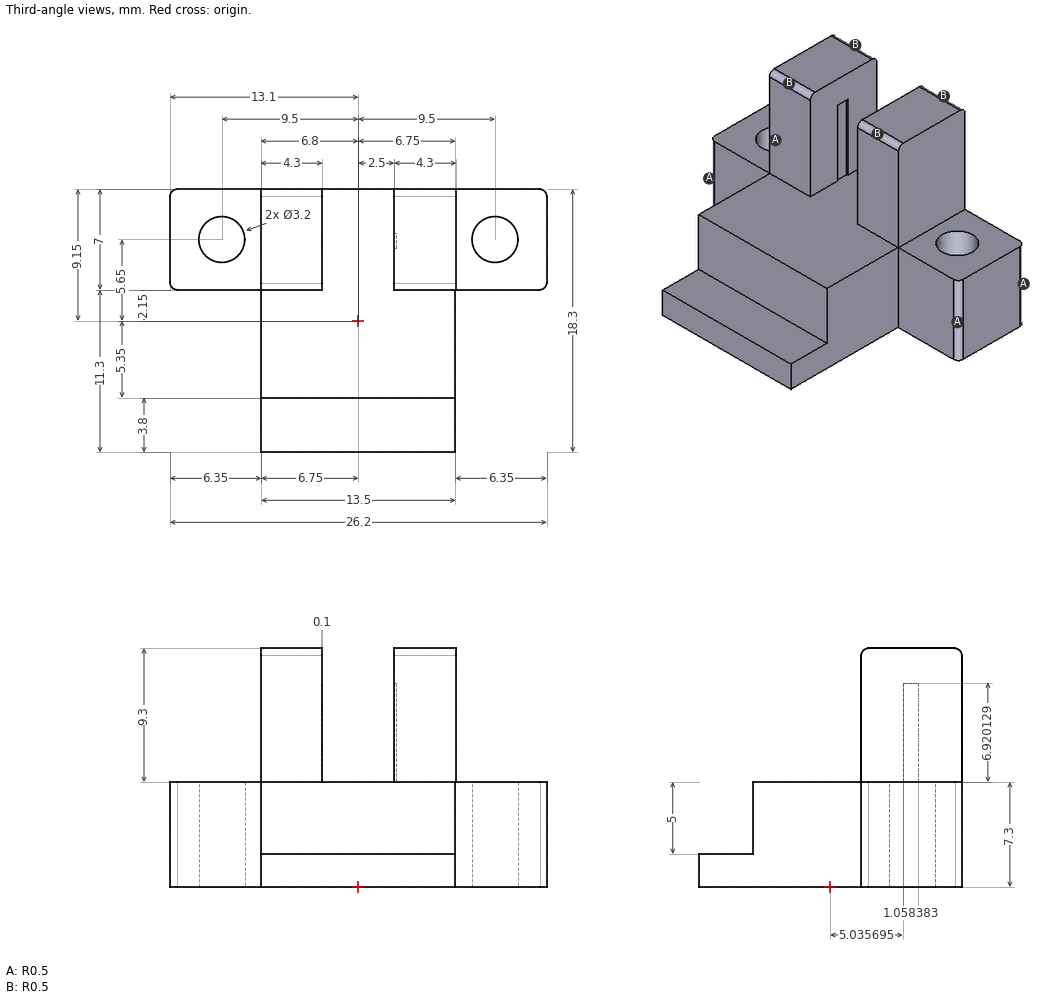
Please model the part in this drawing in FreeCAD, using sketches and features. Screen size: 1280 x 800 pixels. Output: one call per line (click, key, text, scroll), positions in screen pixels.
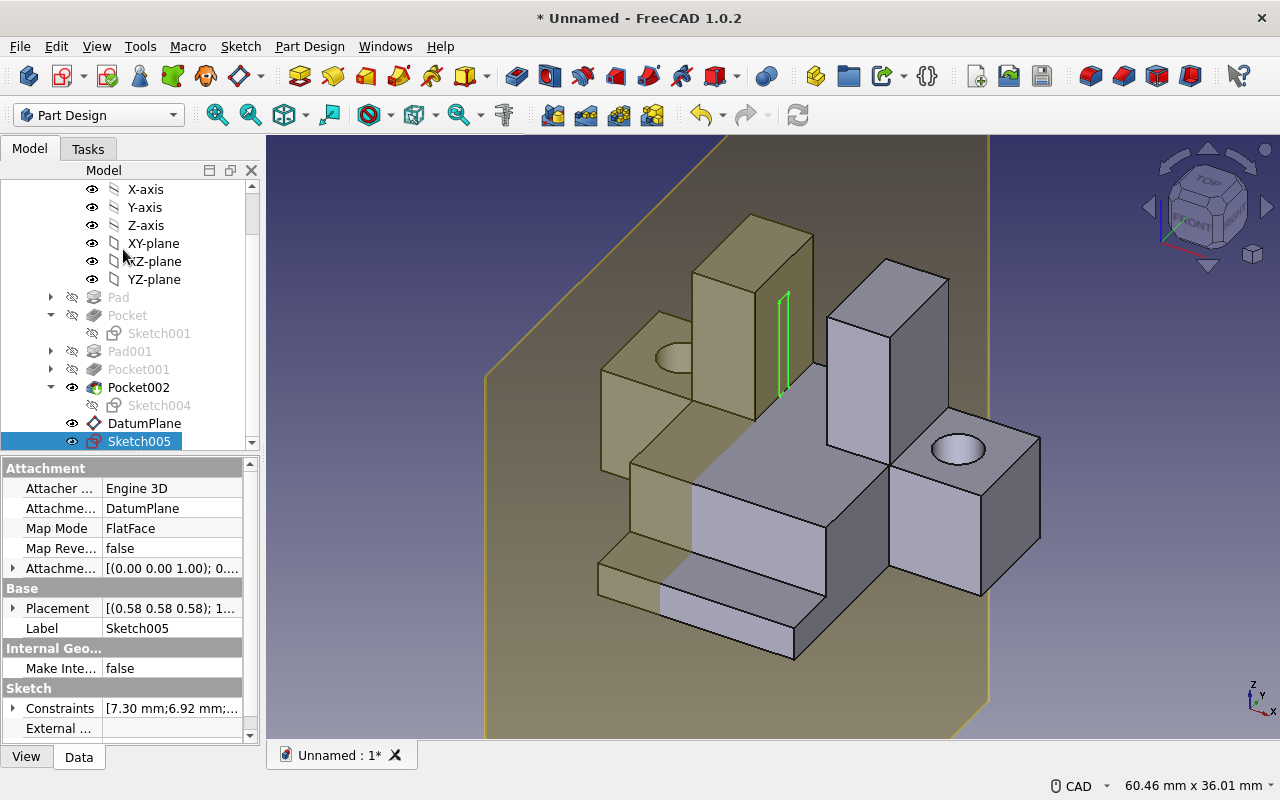
click(517, 76)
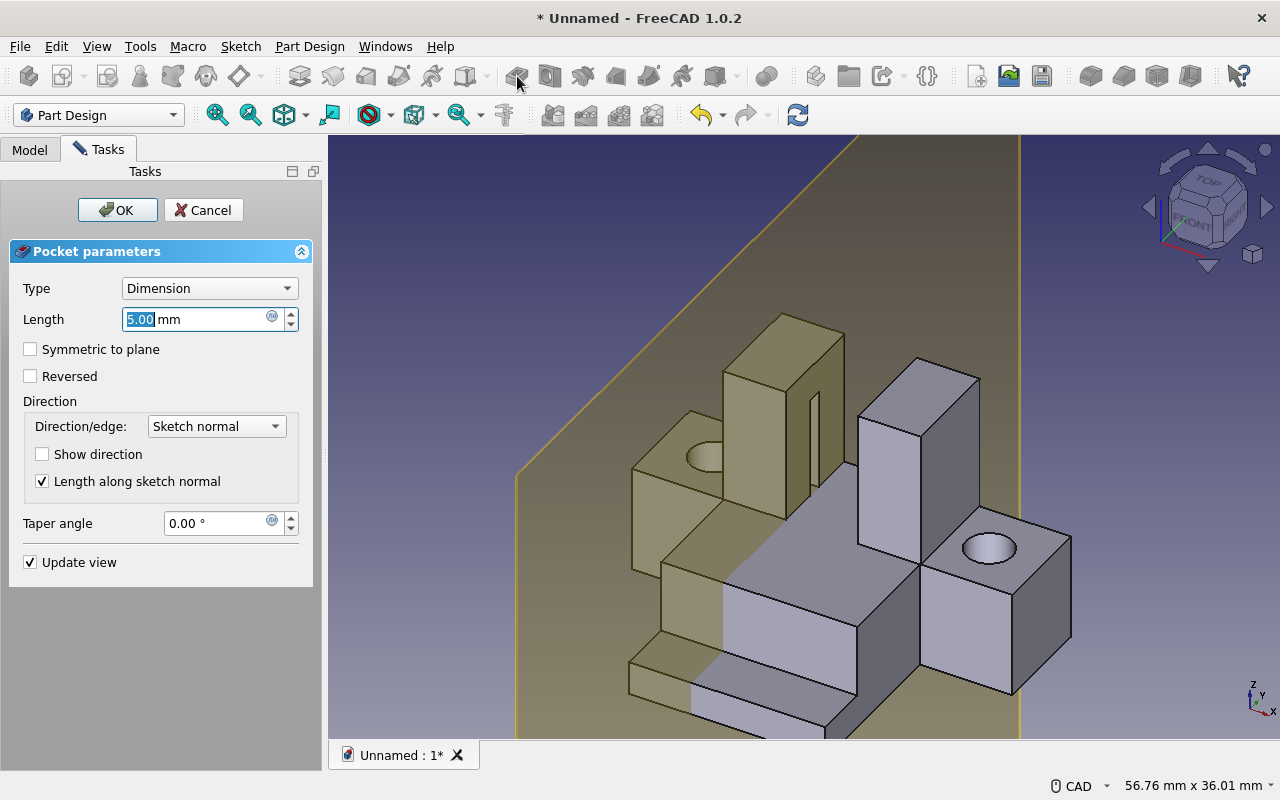
text(0.1)
key(Tab)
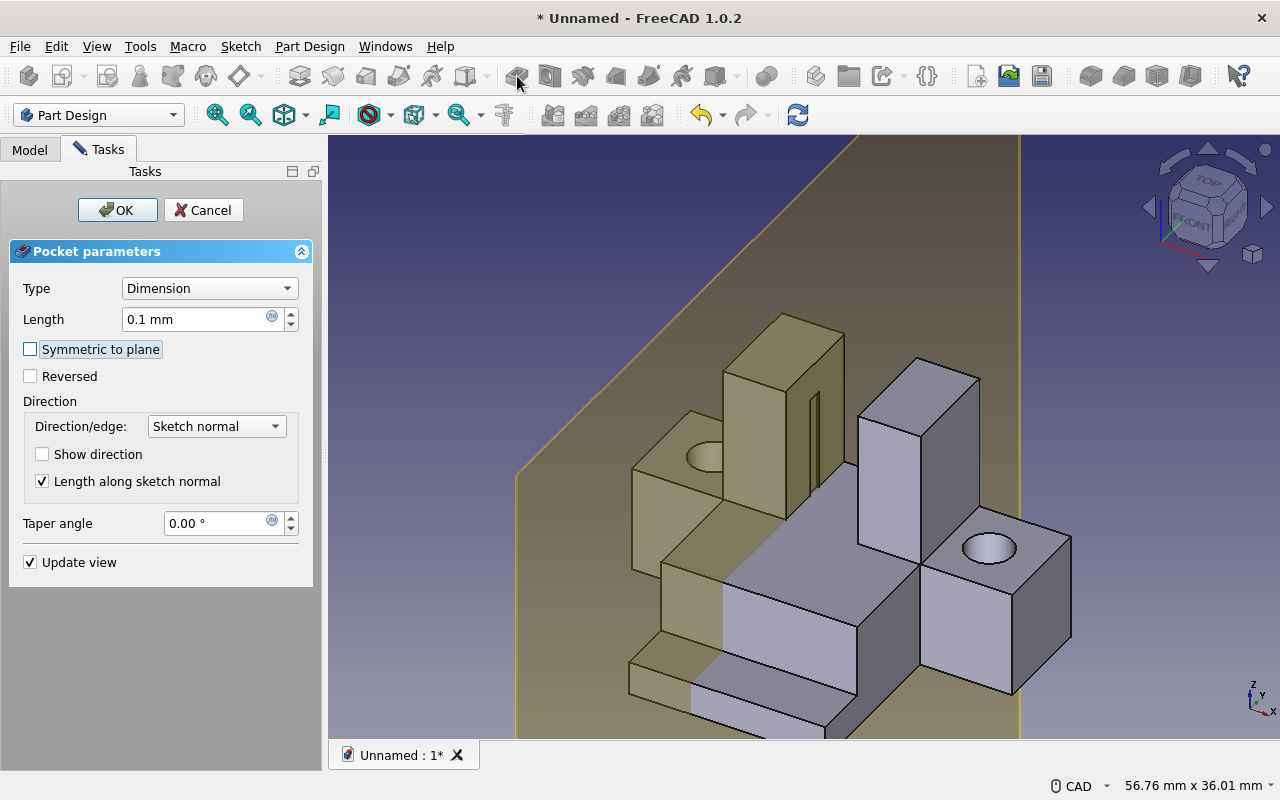
click(118, 210)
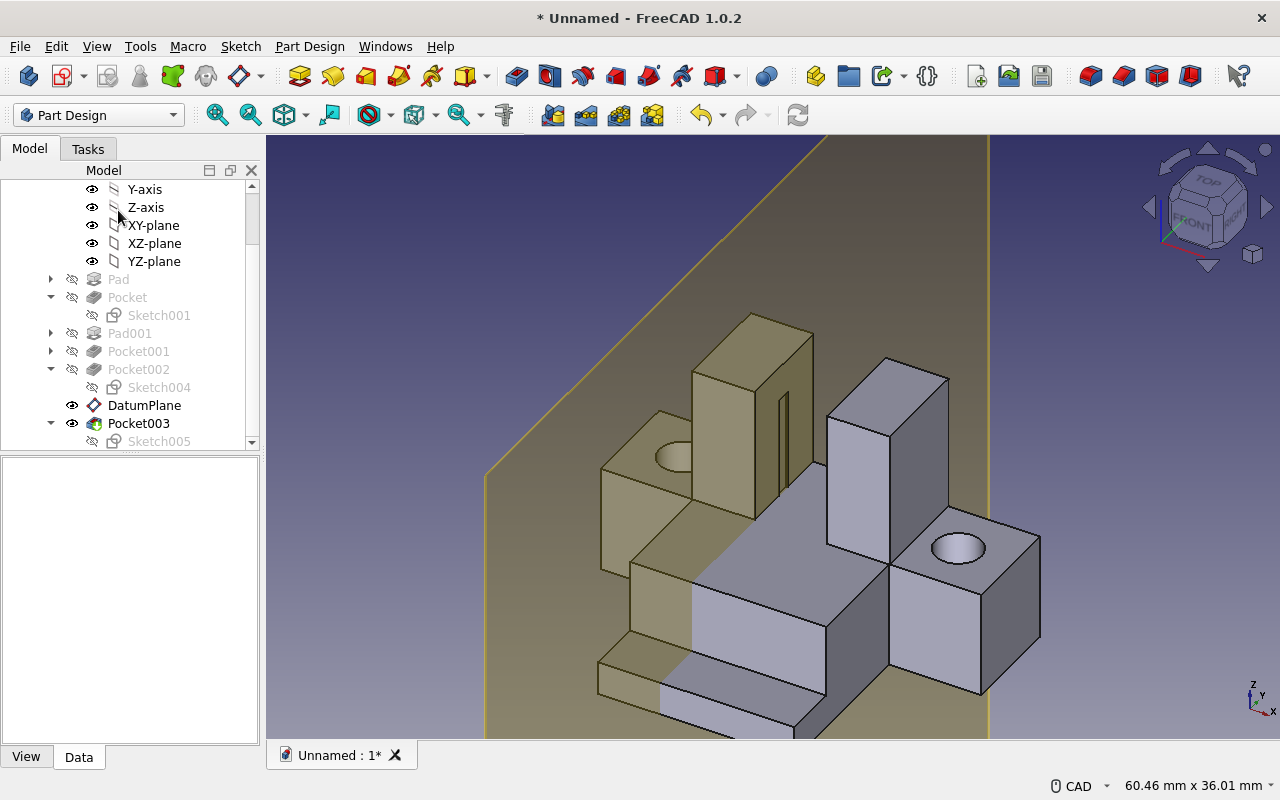
click(117, 405)
key(space)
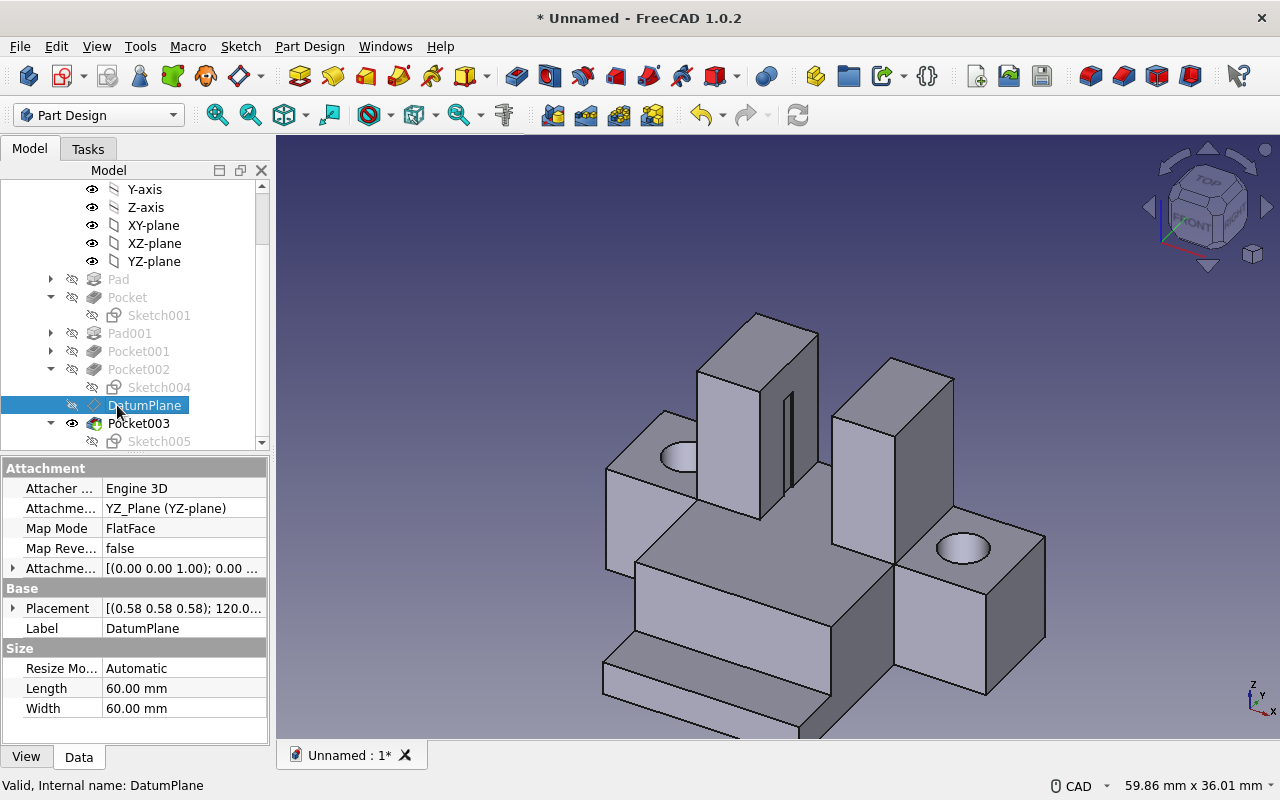
key(v)
key(f)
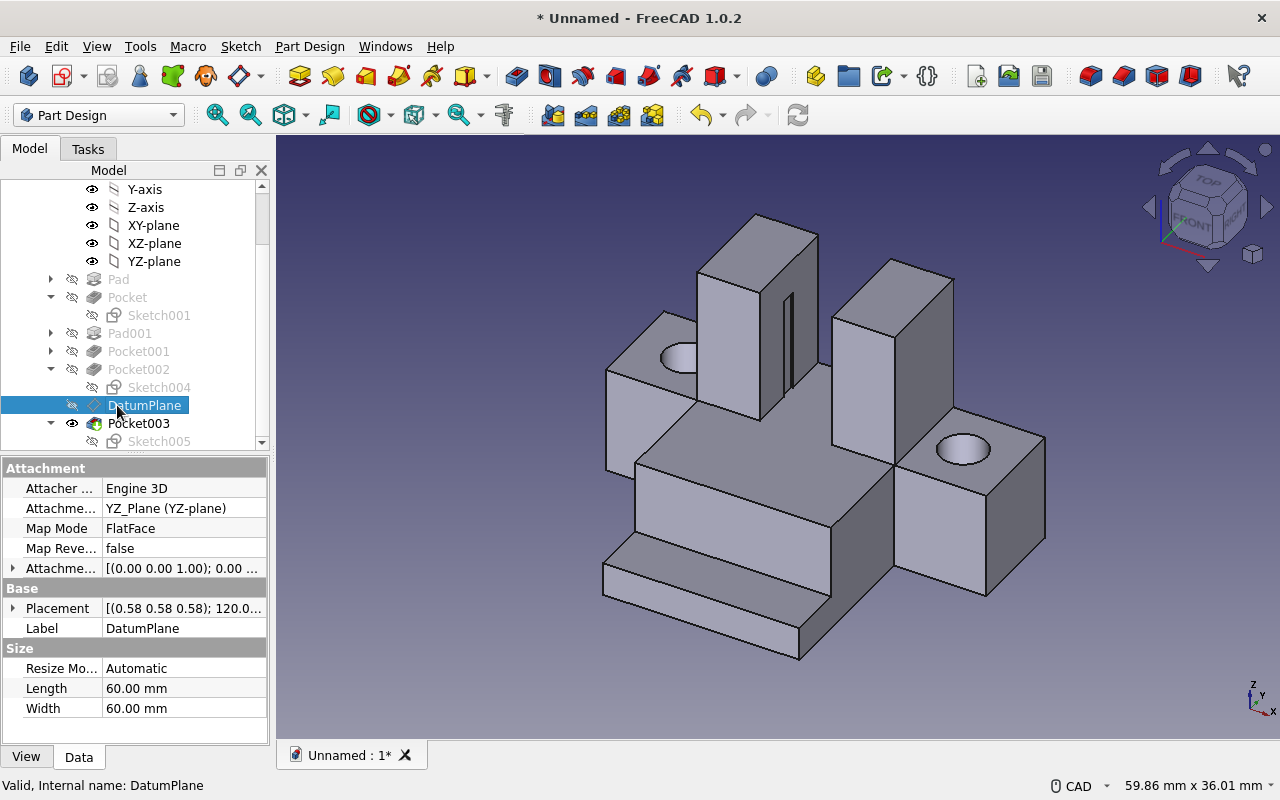
click(986, 545)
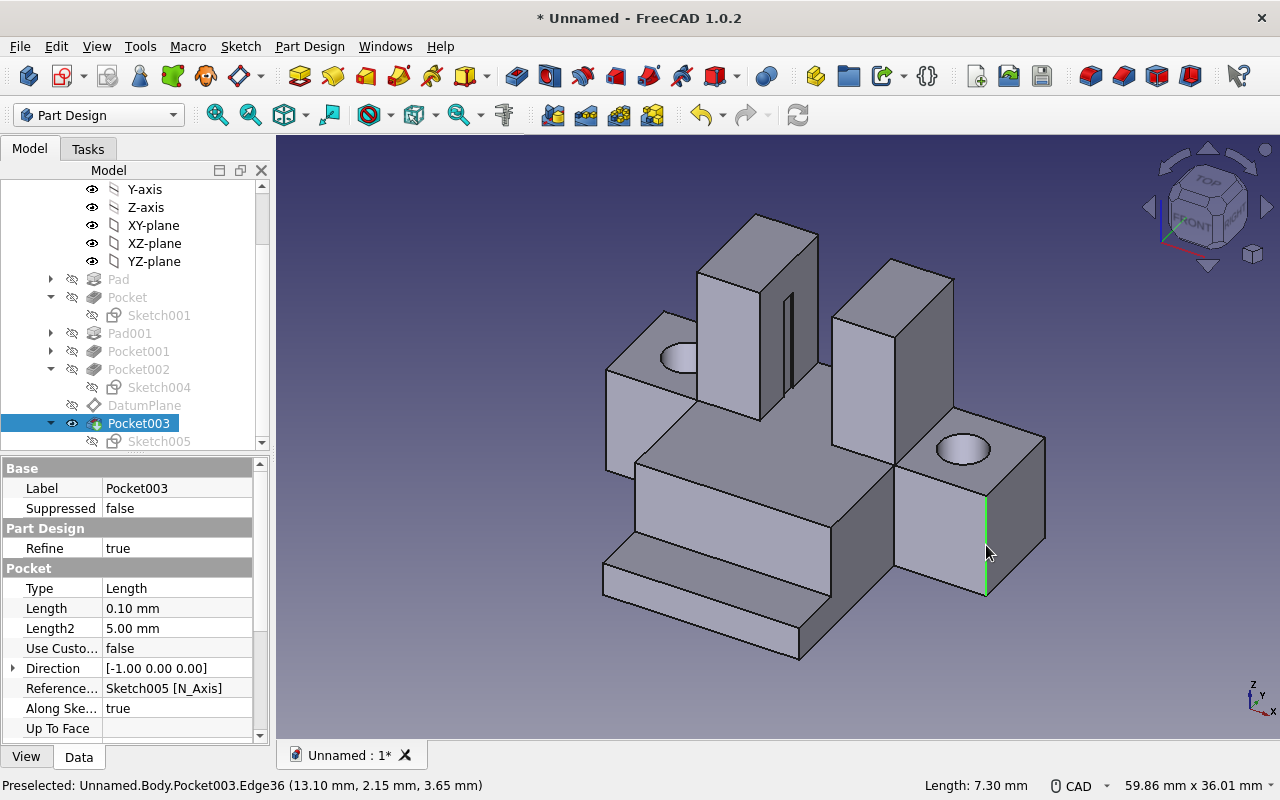
key(0)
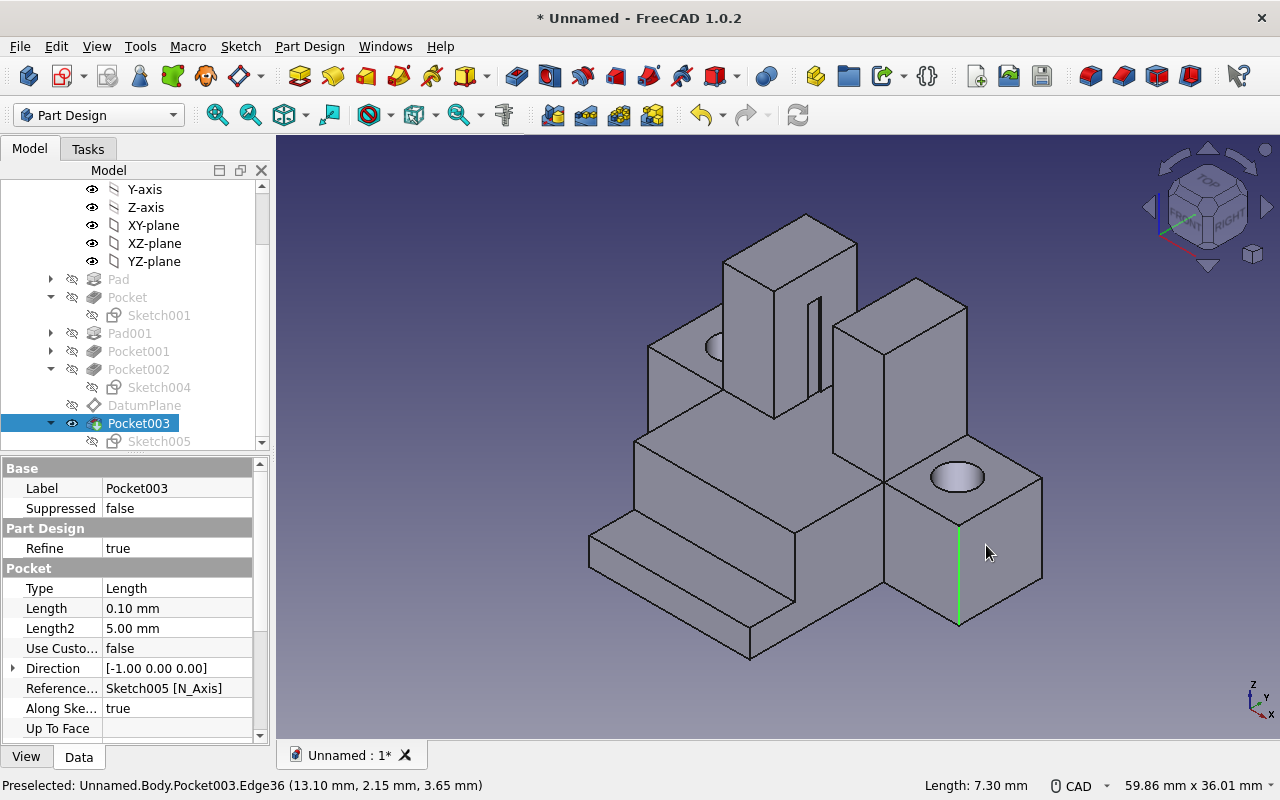
key(2)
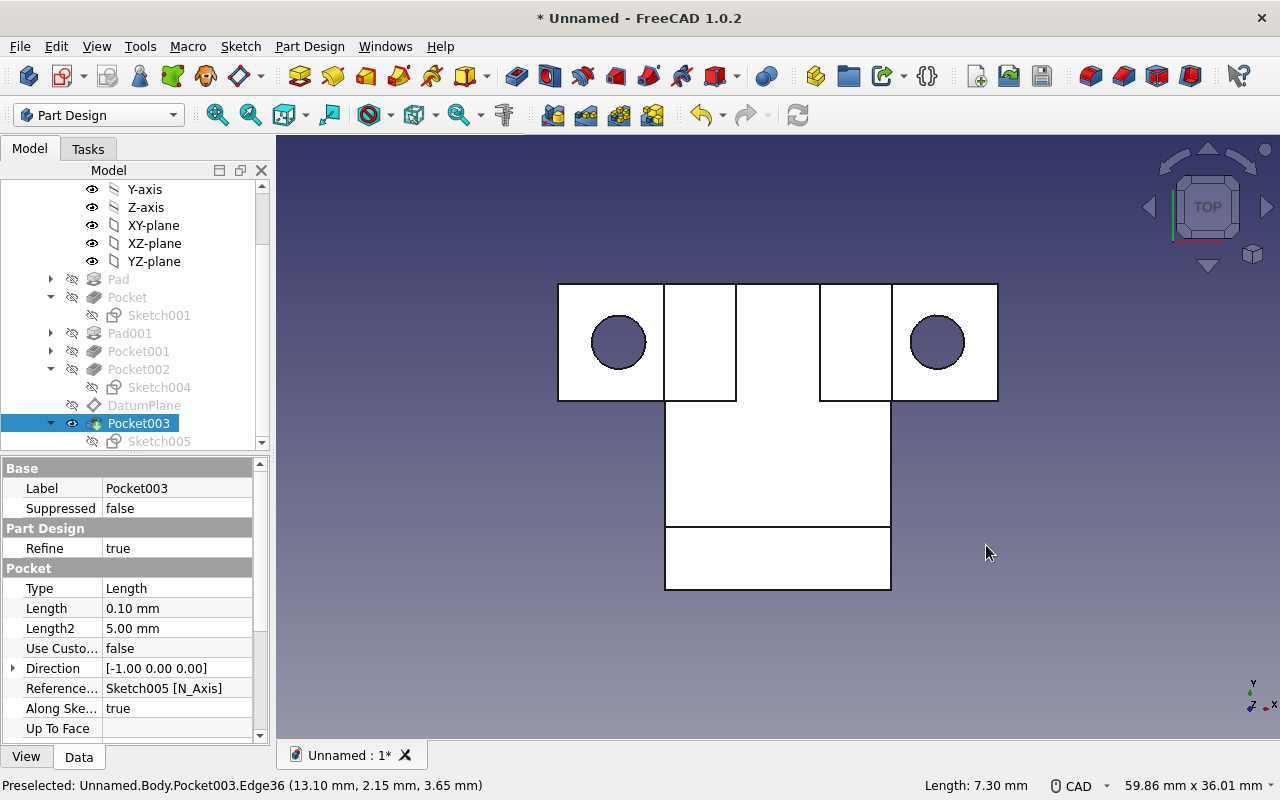
key(1)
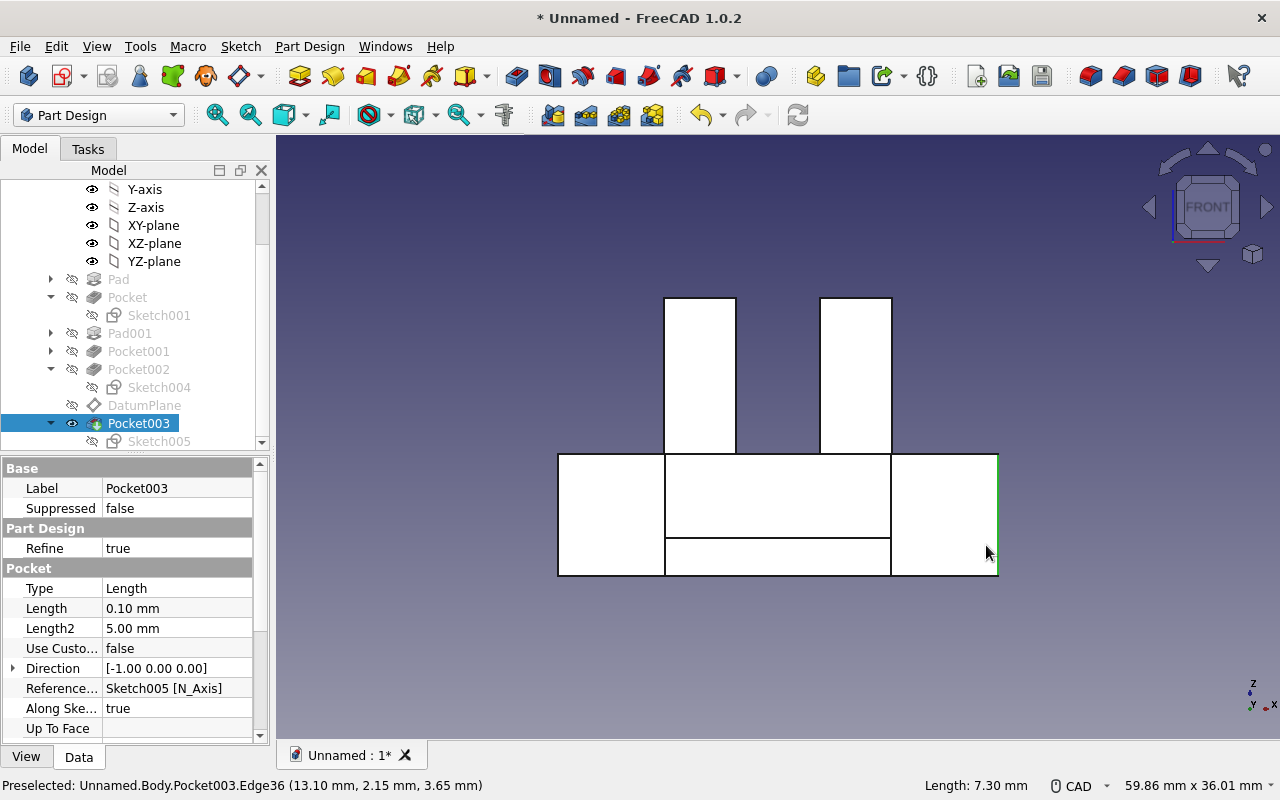
click(558, 514, ctrl)